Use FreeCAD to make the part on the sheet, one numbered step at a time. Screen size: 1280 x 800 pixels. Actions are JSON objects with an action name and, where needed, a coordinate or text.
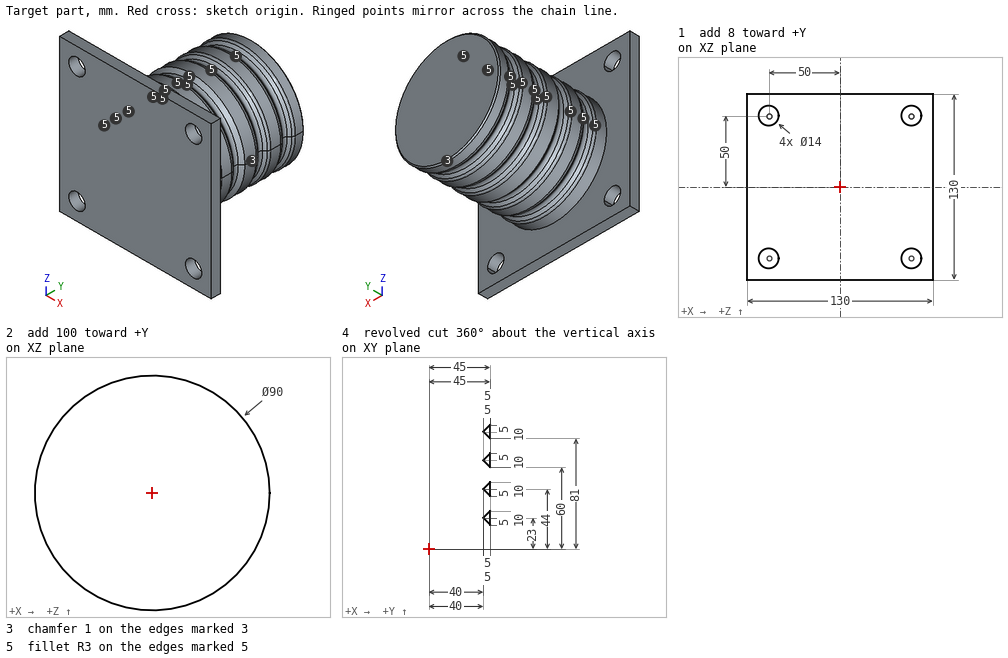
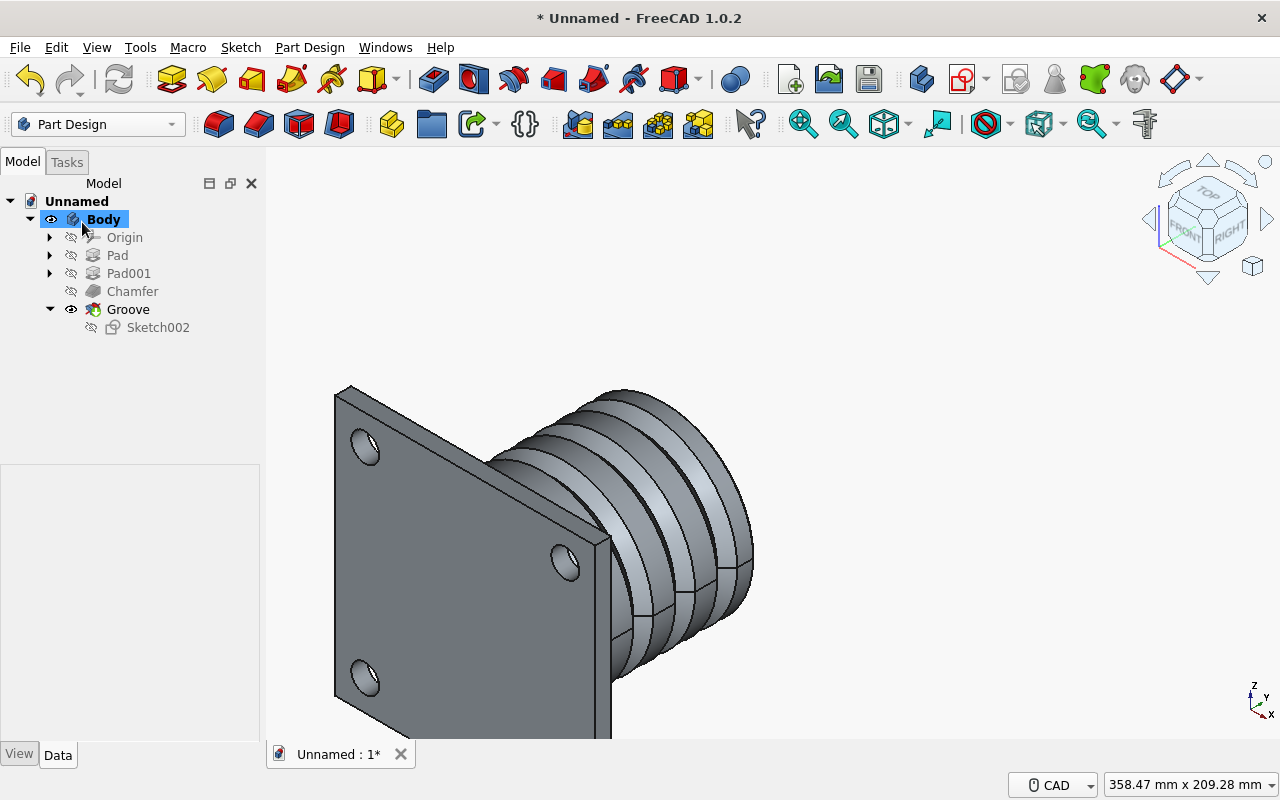
{"action": "left_click", "coordinate": [804, 124]}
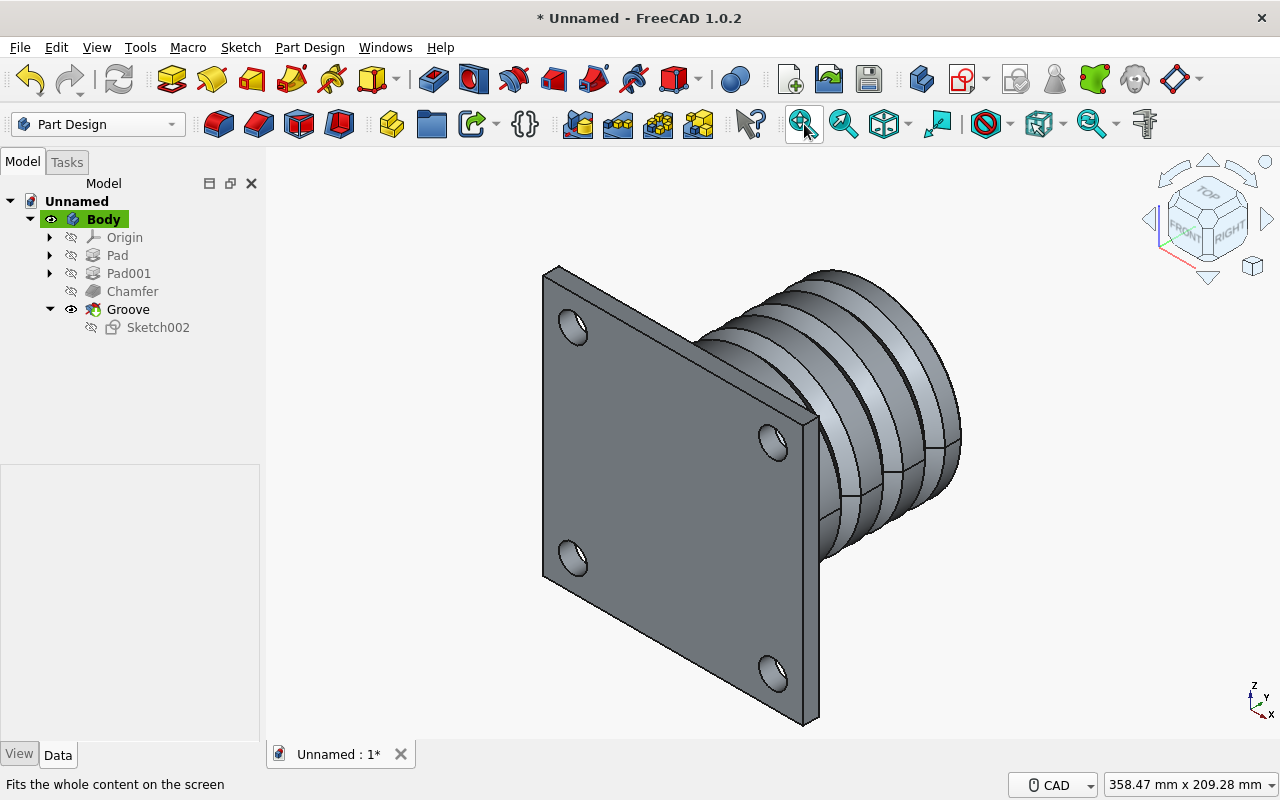
{"action": "left_click", "coordinate": [785, 304]}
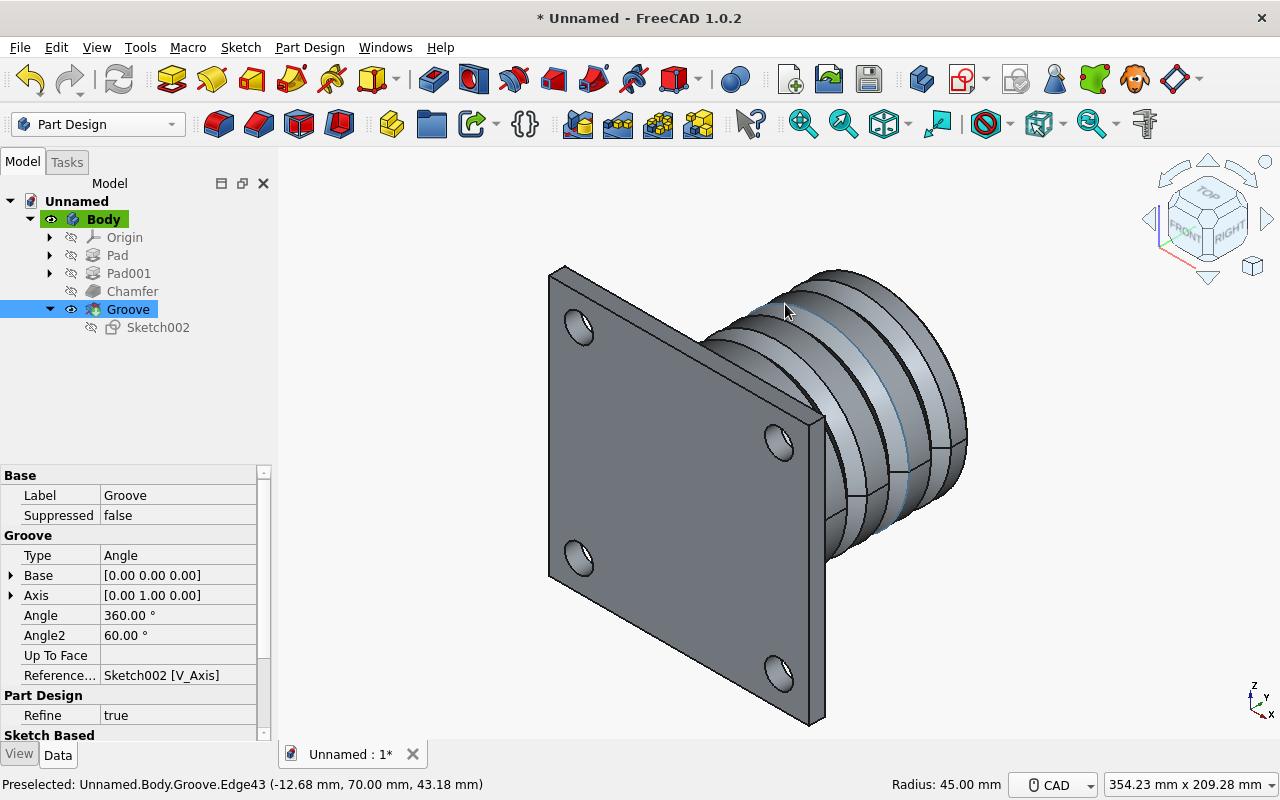
{"action": "left_click", "coordinate": [833, 280], "text": "ctrl"}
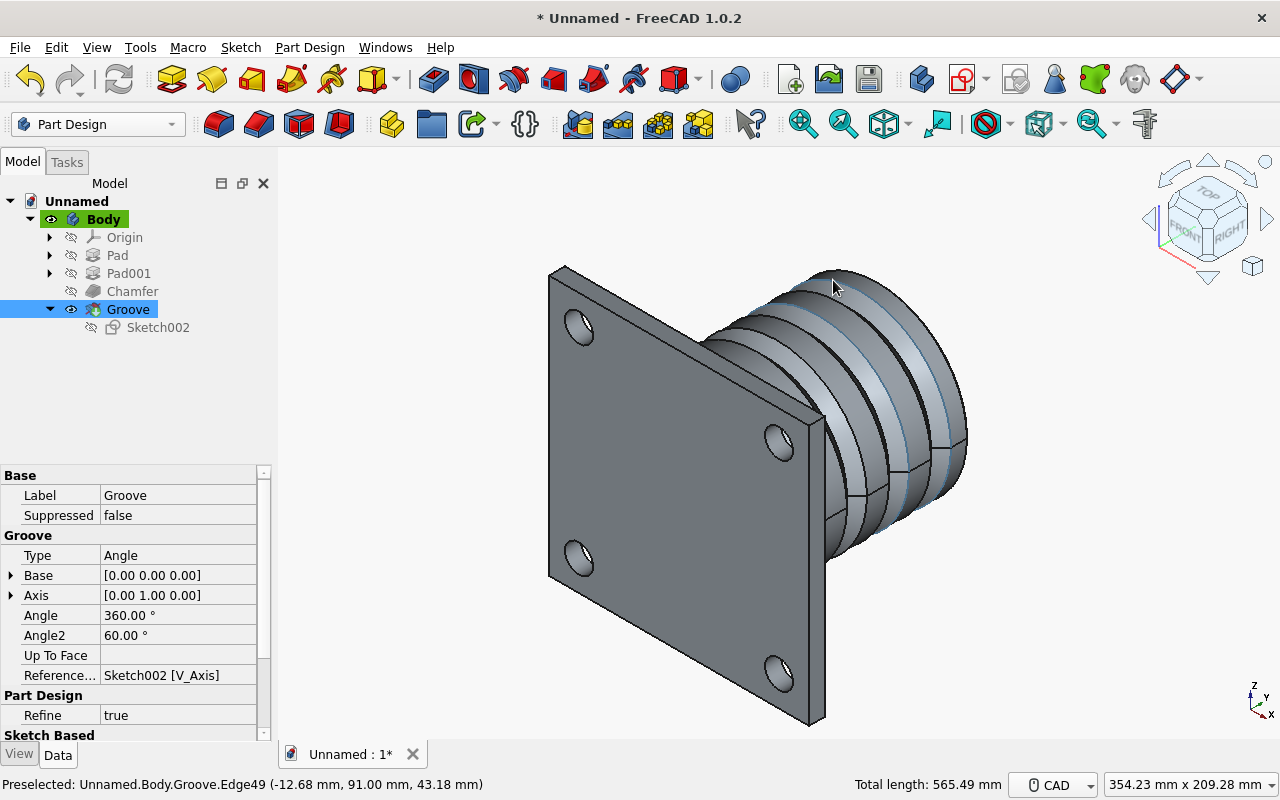
{"action": "left_click", "coordinate": [813, 291], "text": "ctrl"}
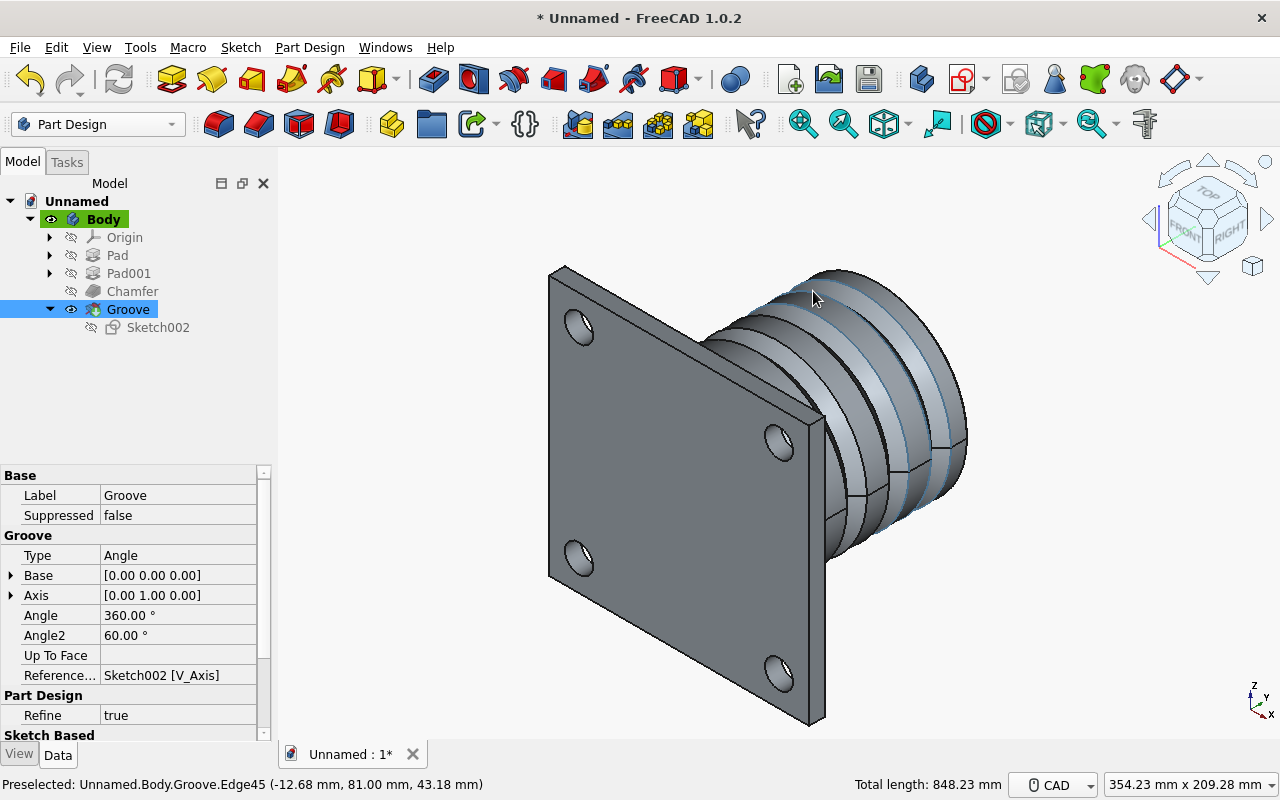
{"action": "key", "text": "2"}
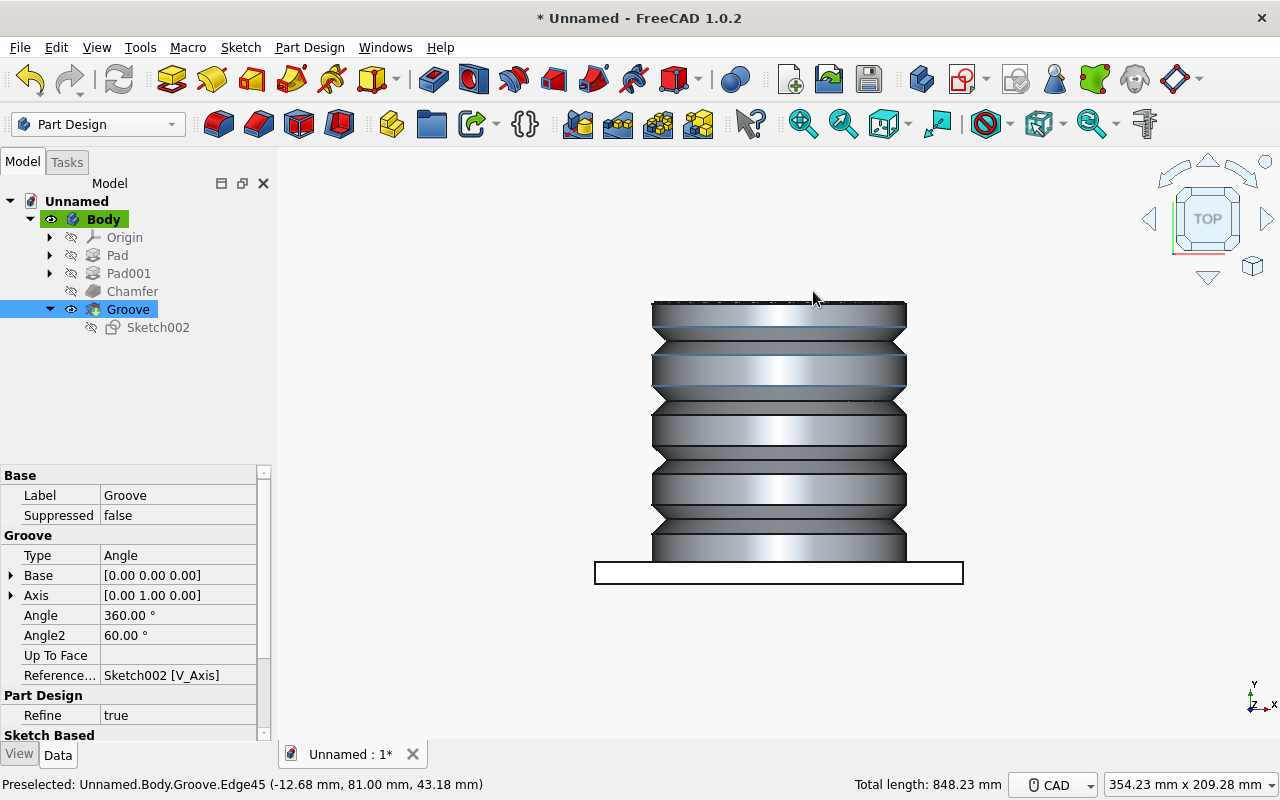
{"action": "left_click", "coordinate": [740, 504], "text": "ctrl"}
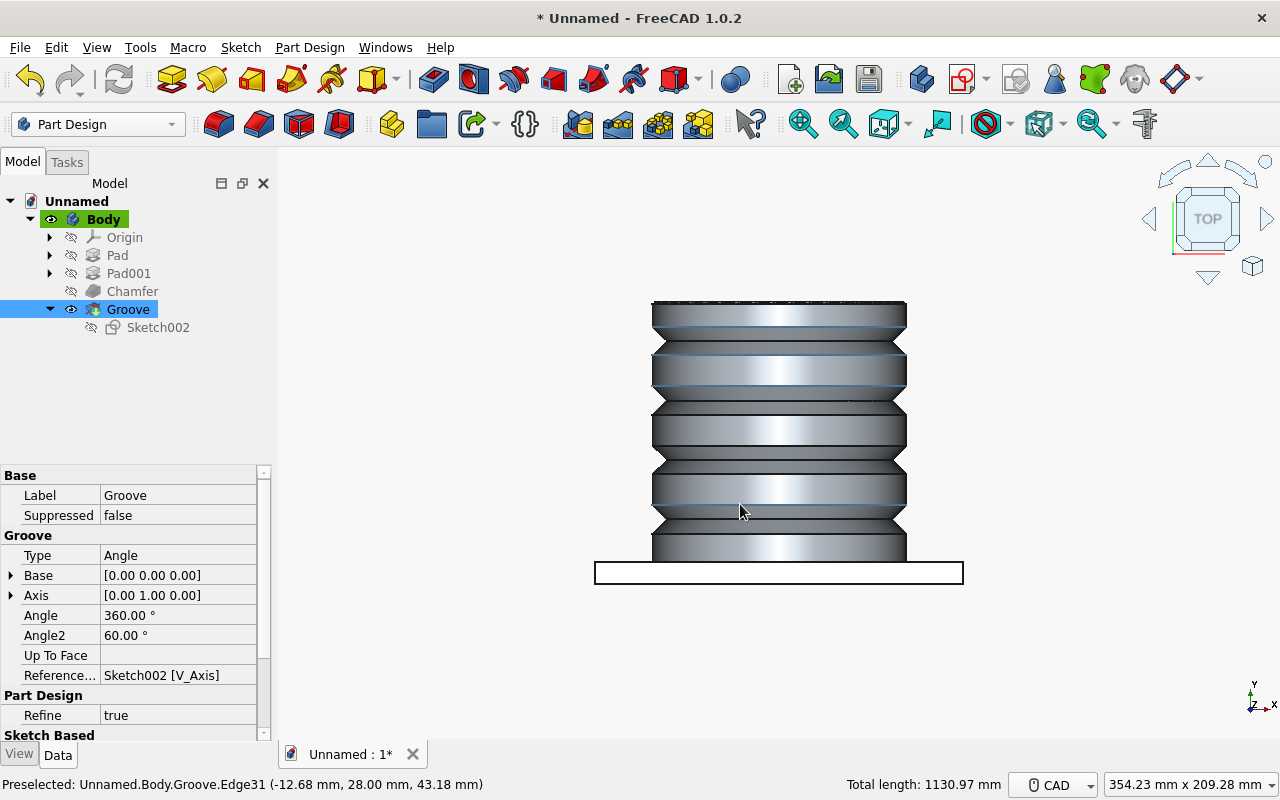
{"action": "left_click", "coordinate": [676, 533], "text": "ctrl"}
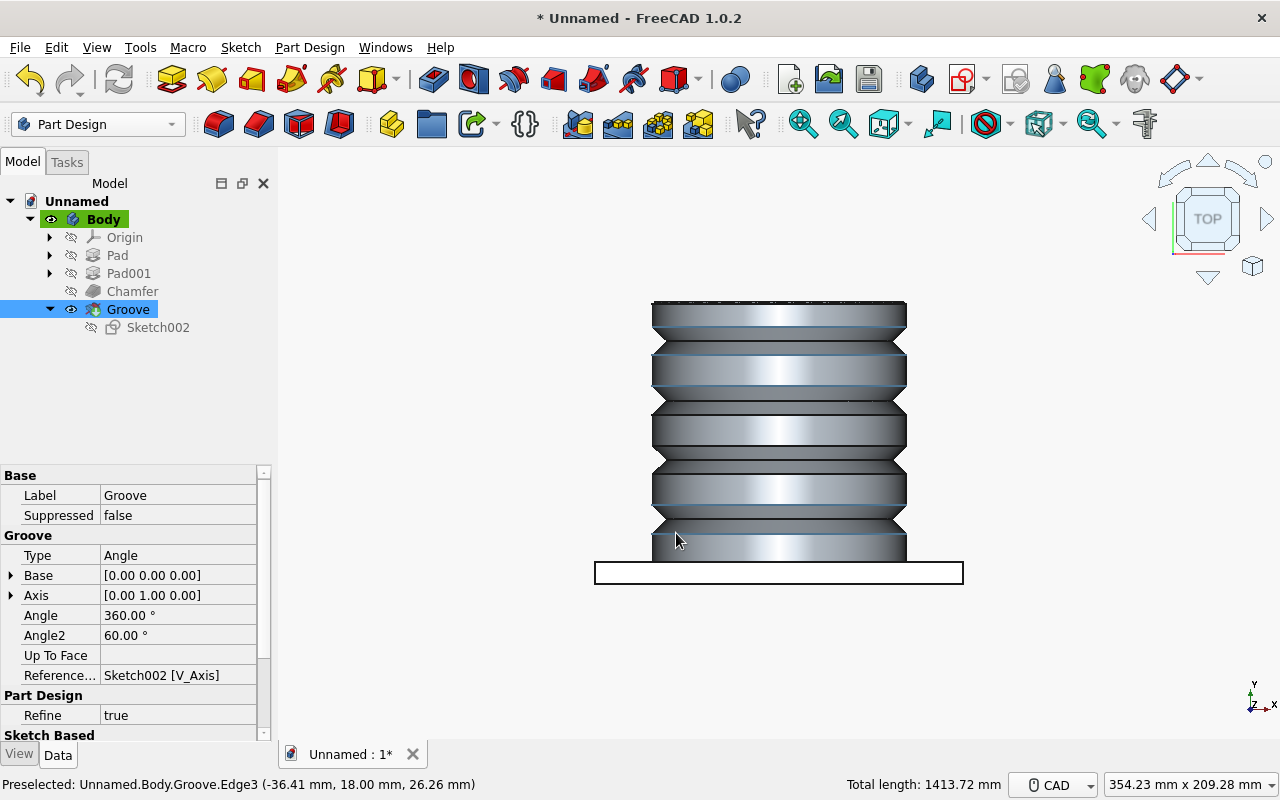
{"action": "left_click", "coordinate": [676, 473], "text": "ctrl"}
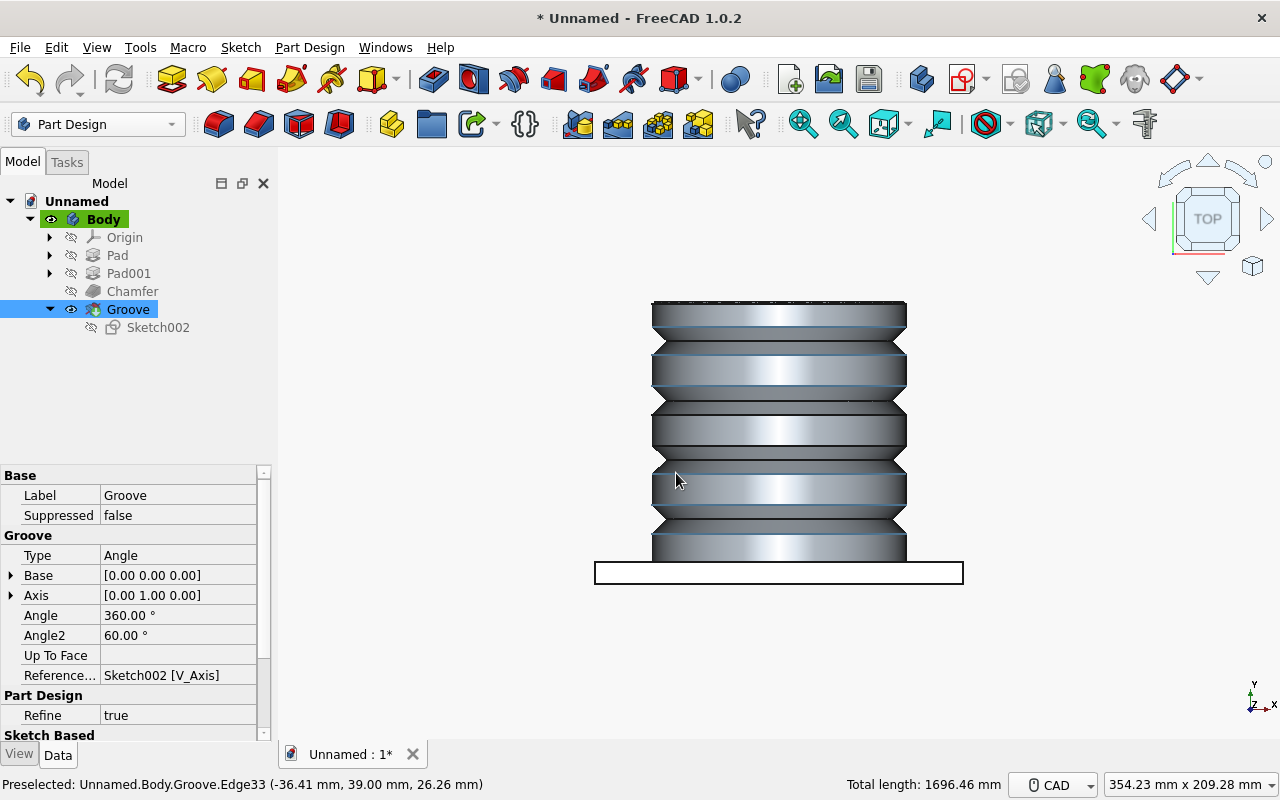
{"action": "left_click", "coordinate": [676, 414], "text": "ctrl"}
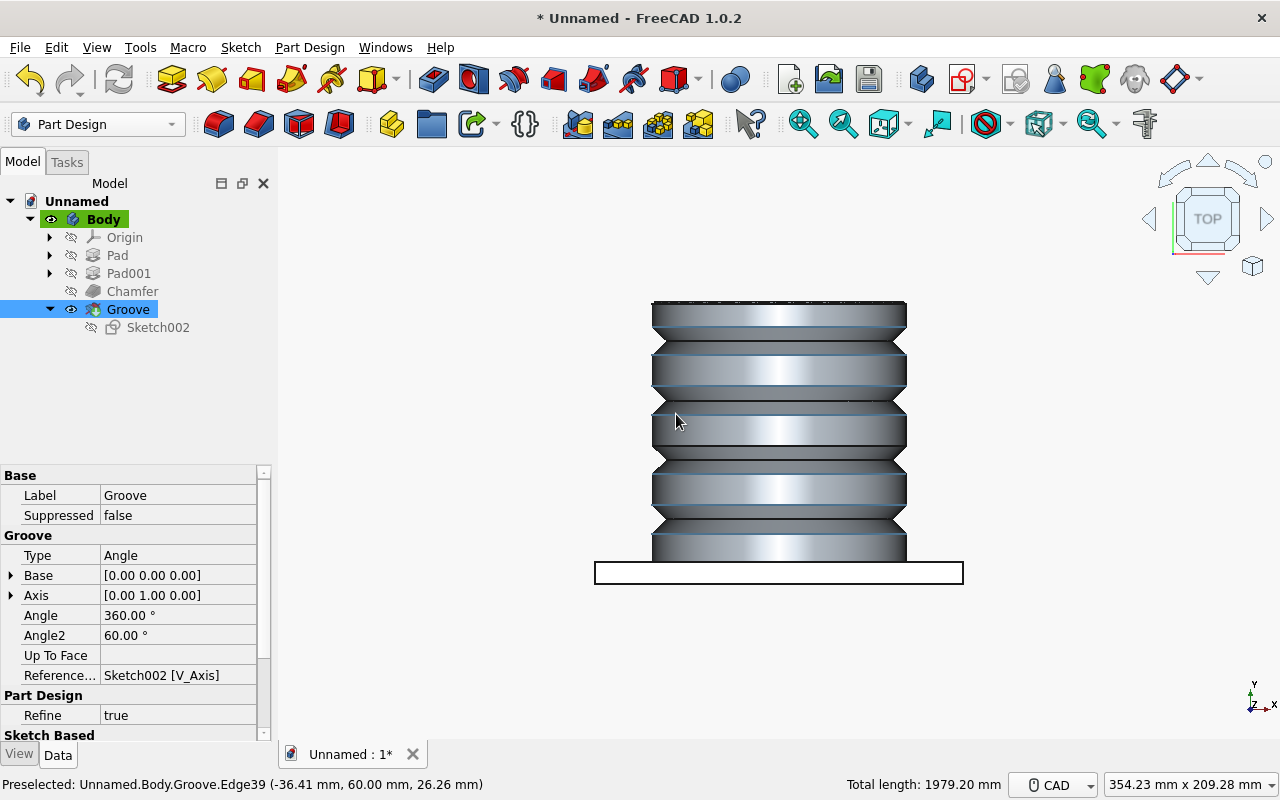
{"action": "key", "text": "0"}